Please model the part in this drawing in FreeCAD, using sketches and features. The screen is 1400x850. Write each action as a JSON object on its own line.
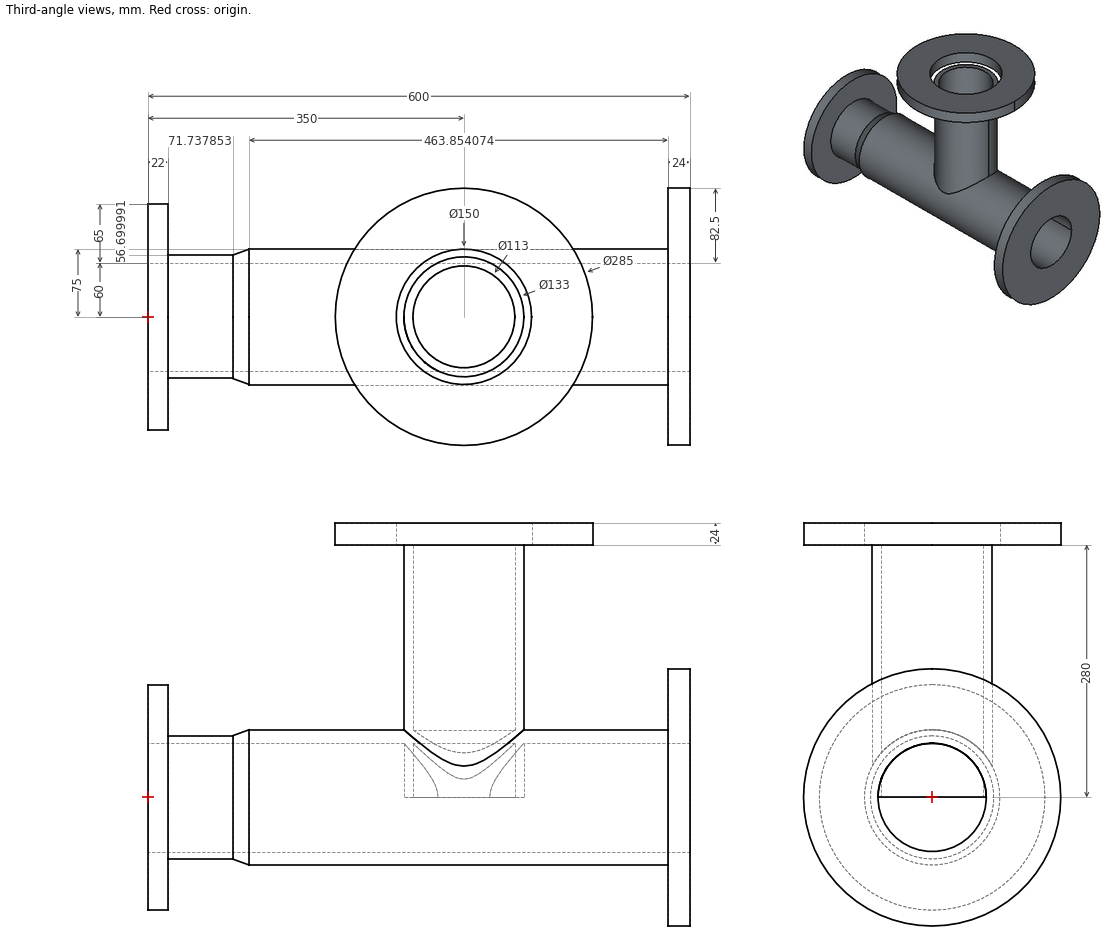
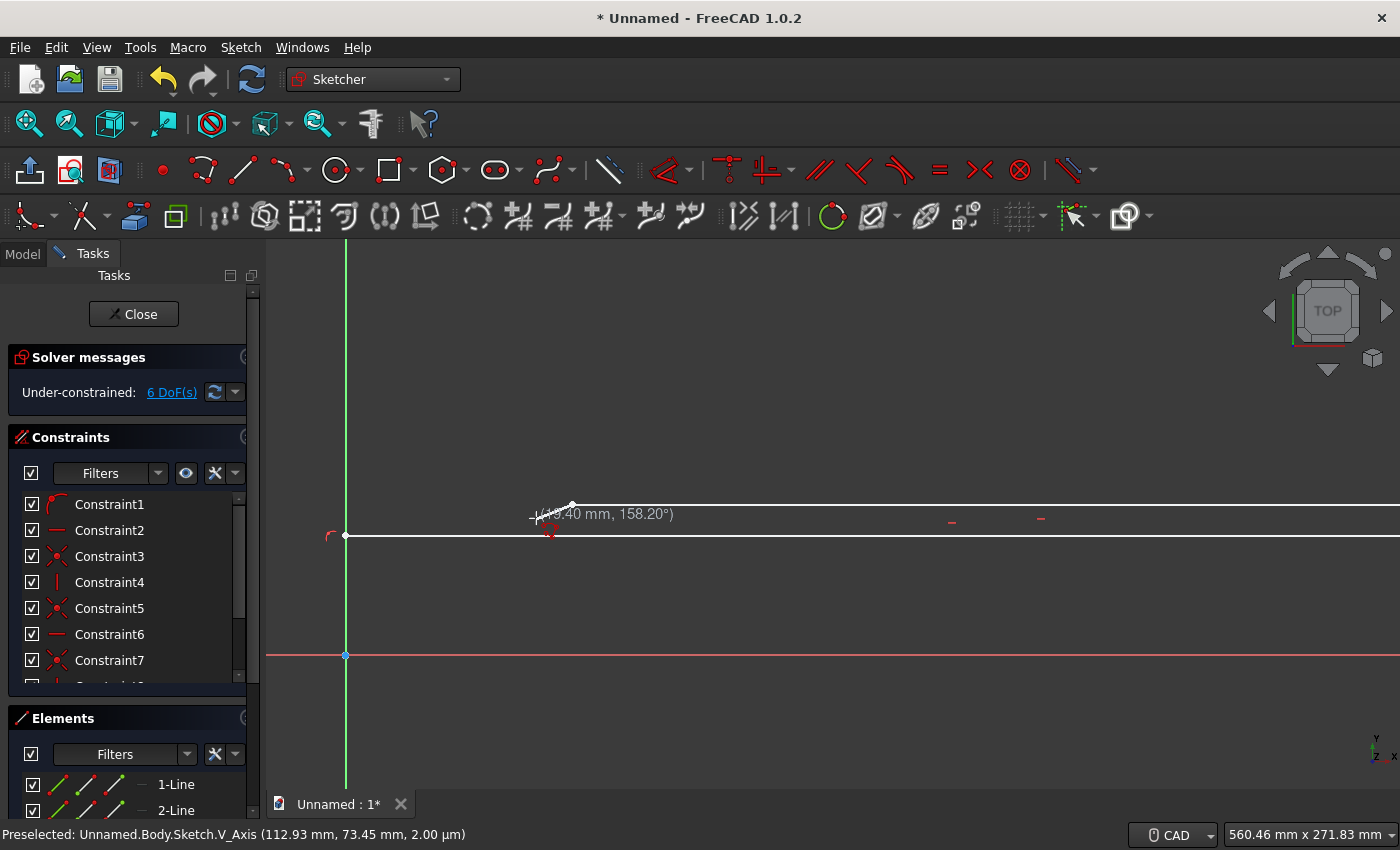
{"action": "left_click", "coordinate": [535, 517]}
{"action": "left_click", "coordinate": [390, 517]}
{"action": "left_click", "coordinate": [390, 402]}
{"action": "left_click", "coordinate": [355, 402]}
{"action": "left_click", "coordinate": [346, 536]}
{"action": "key", "text": "Escape"}
{"action": "key", "text": "Escape"}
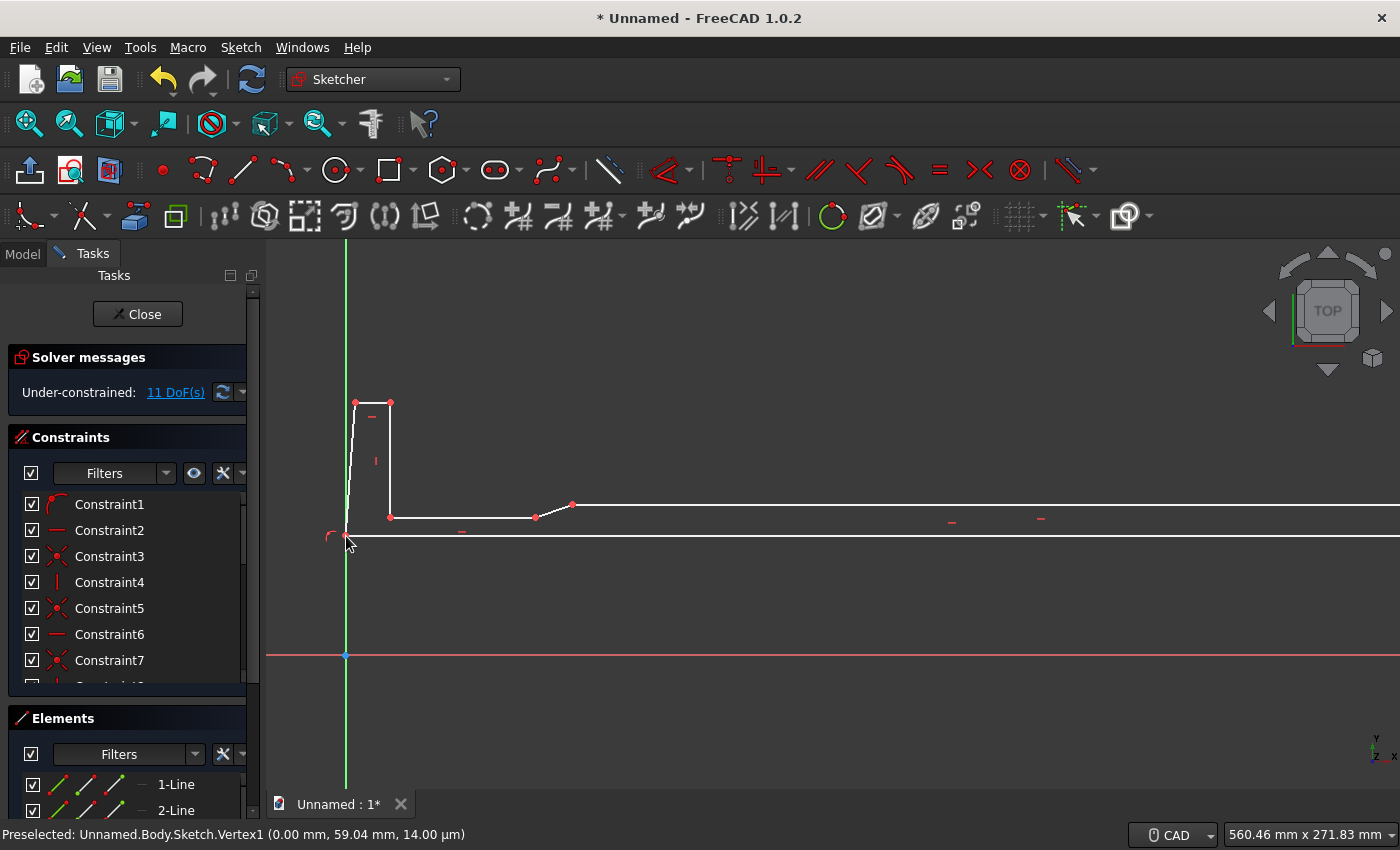
{"action": "left_click", "coordinate": [348, 496]}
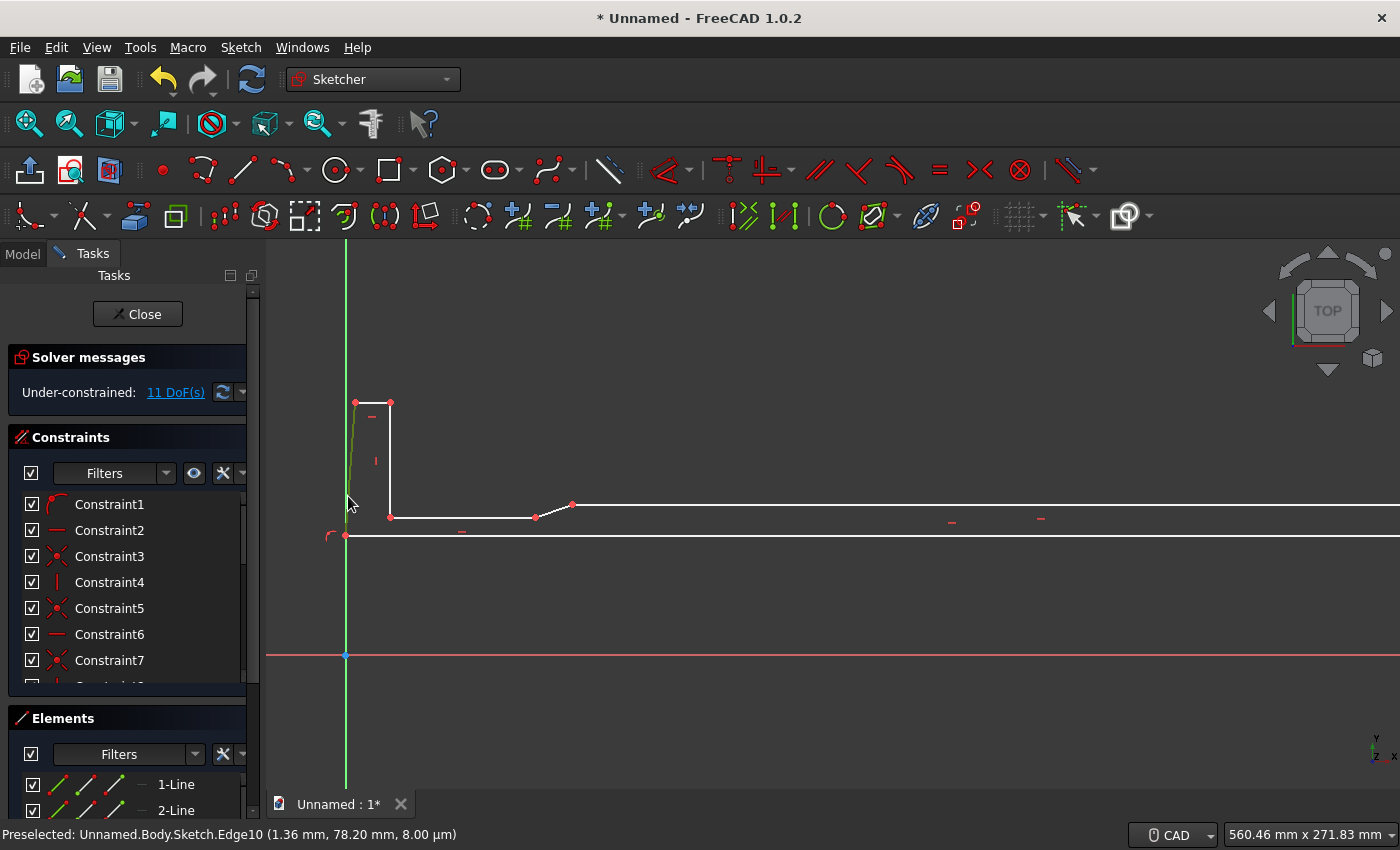
{"action": "key", "text": "v"}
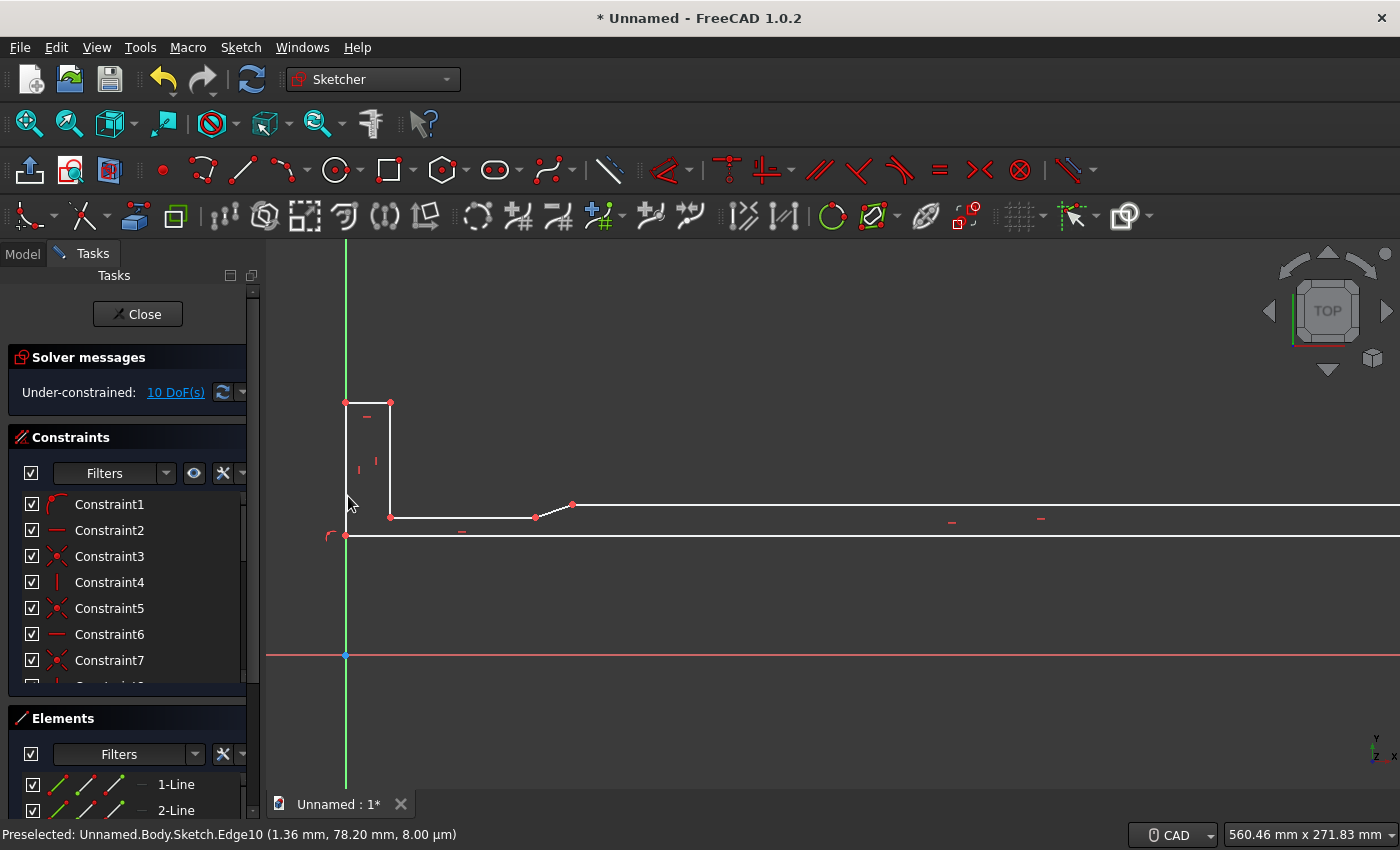
{"action": "left_click", "coordinate": [664, 170]}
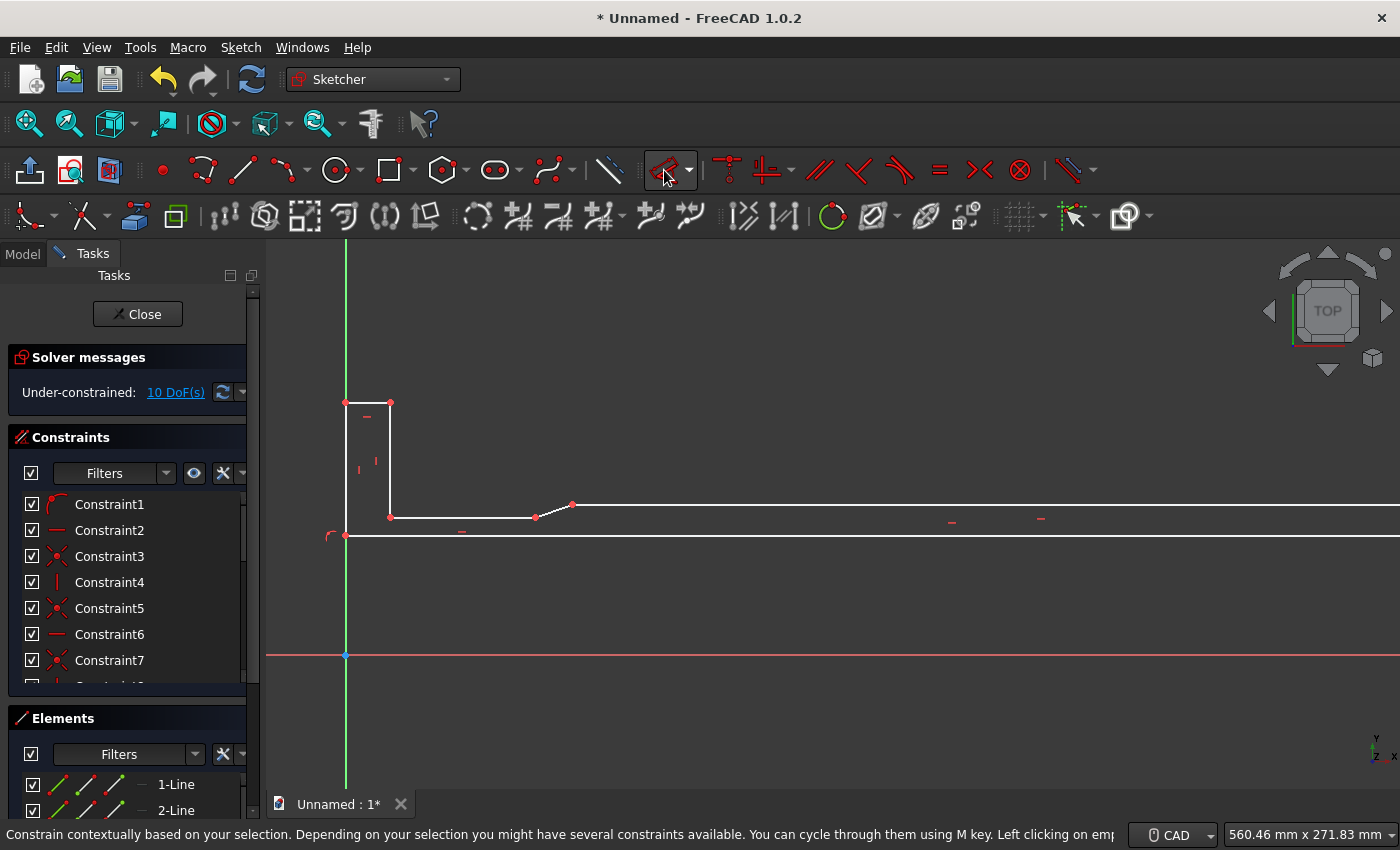
{"action": "scroll", "coordinate": [536, 518], "scroll_direction": "down", "scroll_amount": 3}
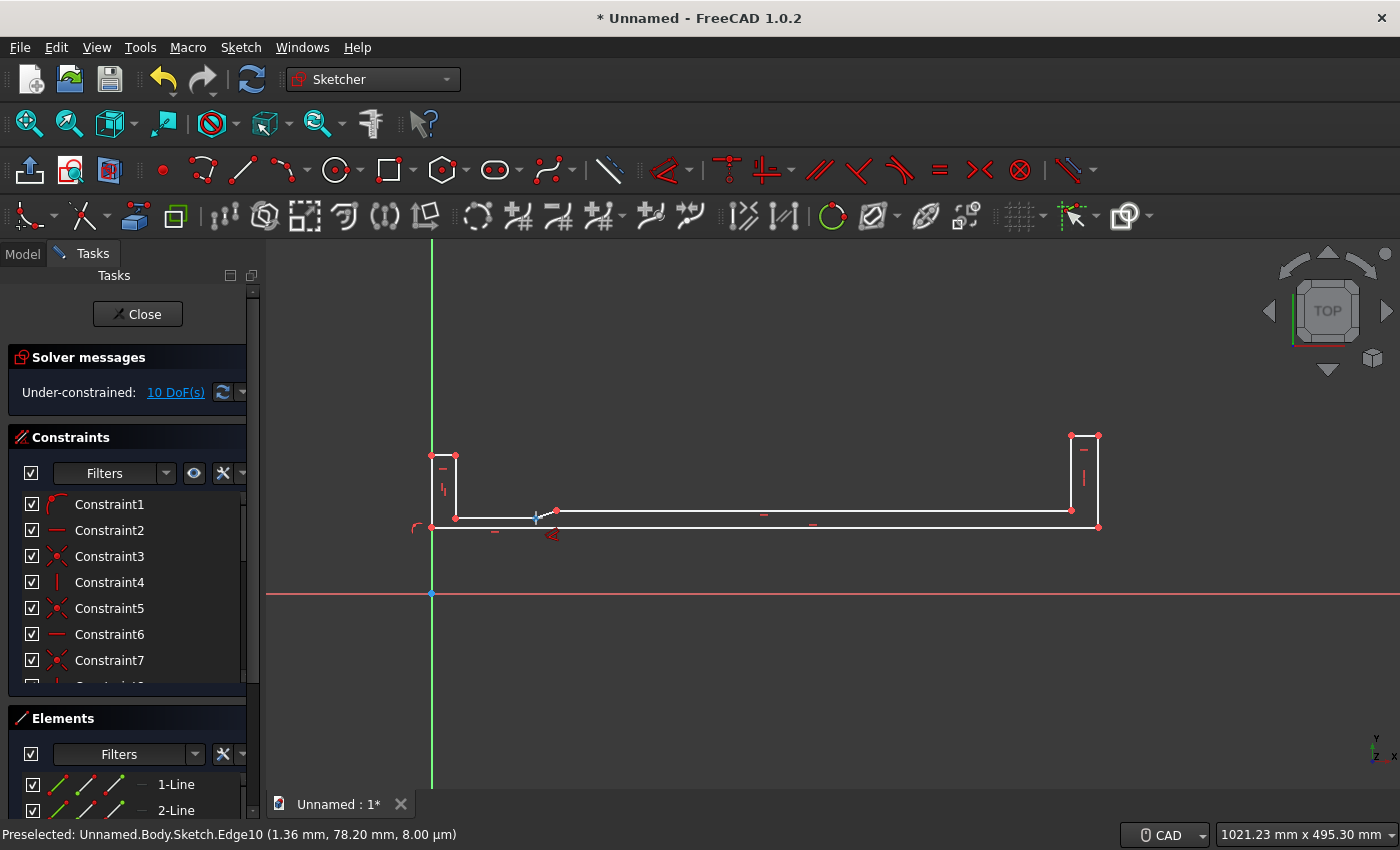
{"action": "scroll", "coordinate": [1090, 436], "scroll_direction": "up", "scroll_amount": 3}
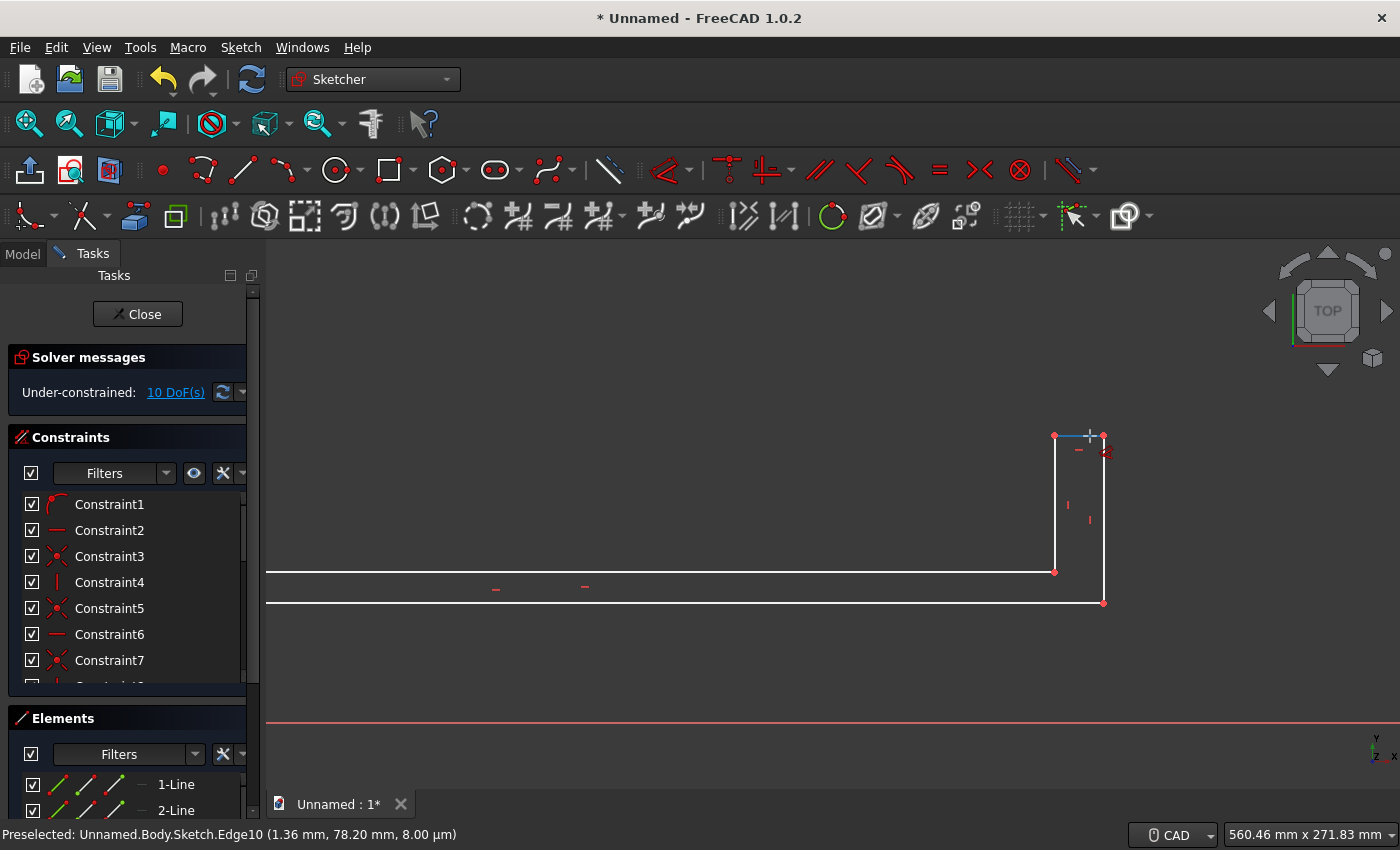
{"action": "left_click", "coordinate": [1089, 436]}
{"action": "left_click", "coordinate": [1079, 402]}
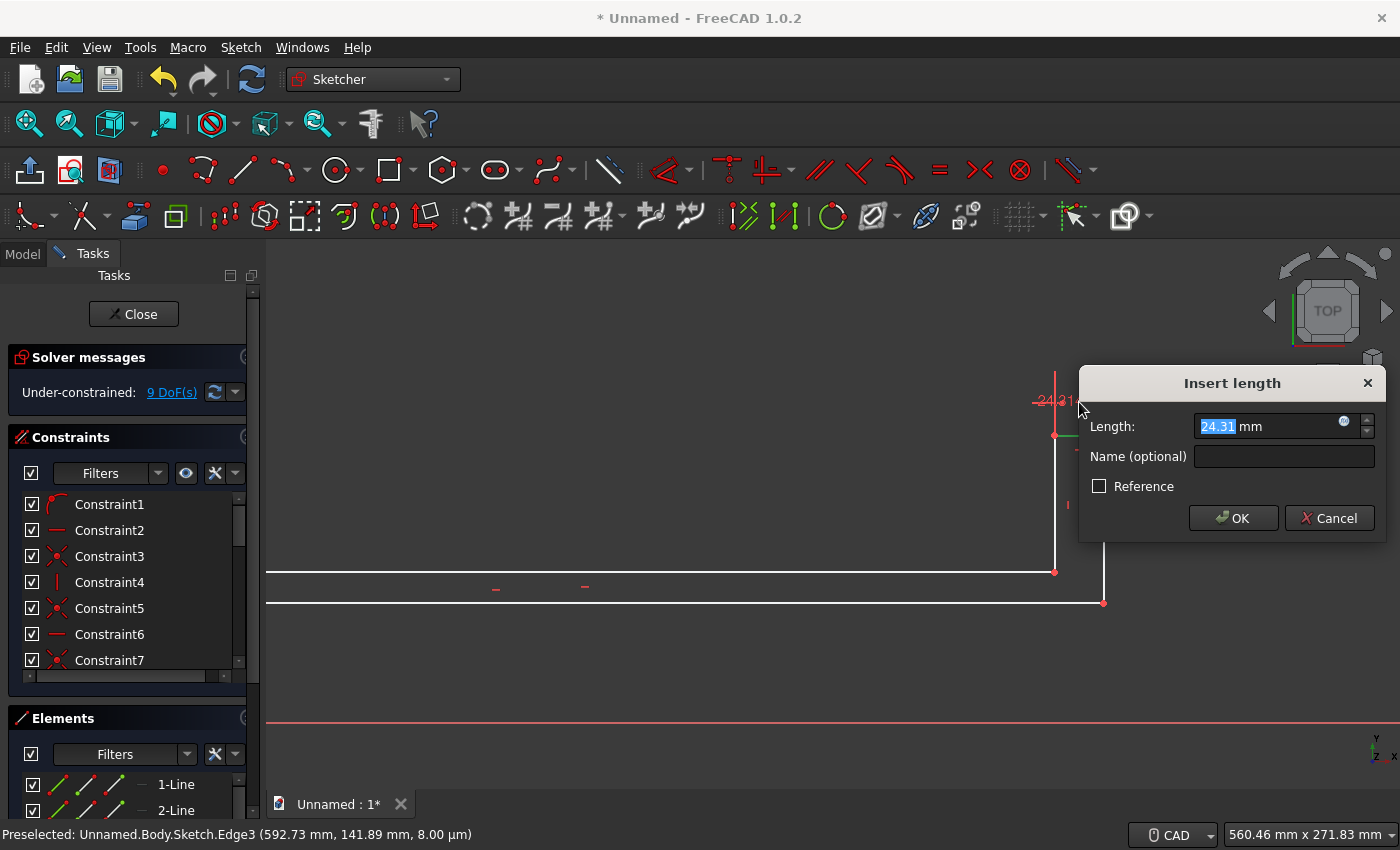
{"action": "type", "text": "24"}
{"action": "key", "text": "Return"}